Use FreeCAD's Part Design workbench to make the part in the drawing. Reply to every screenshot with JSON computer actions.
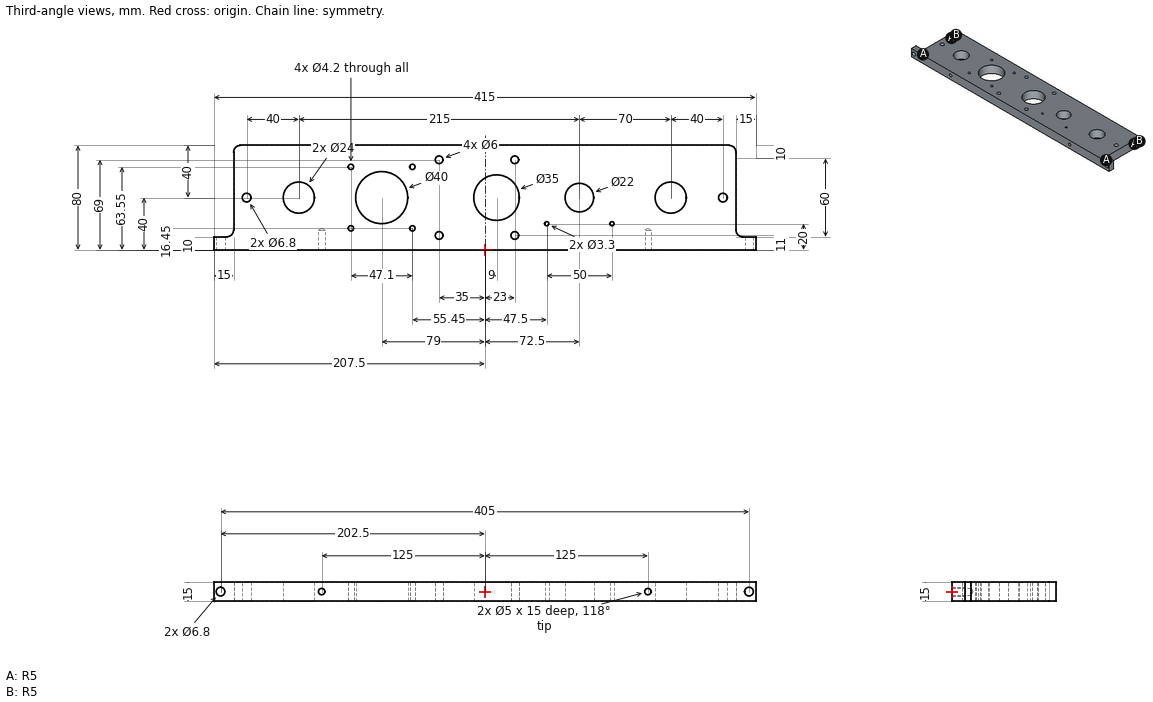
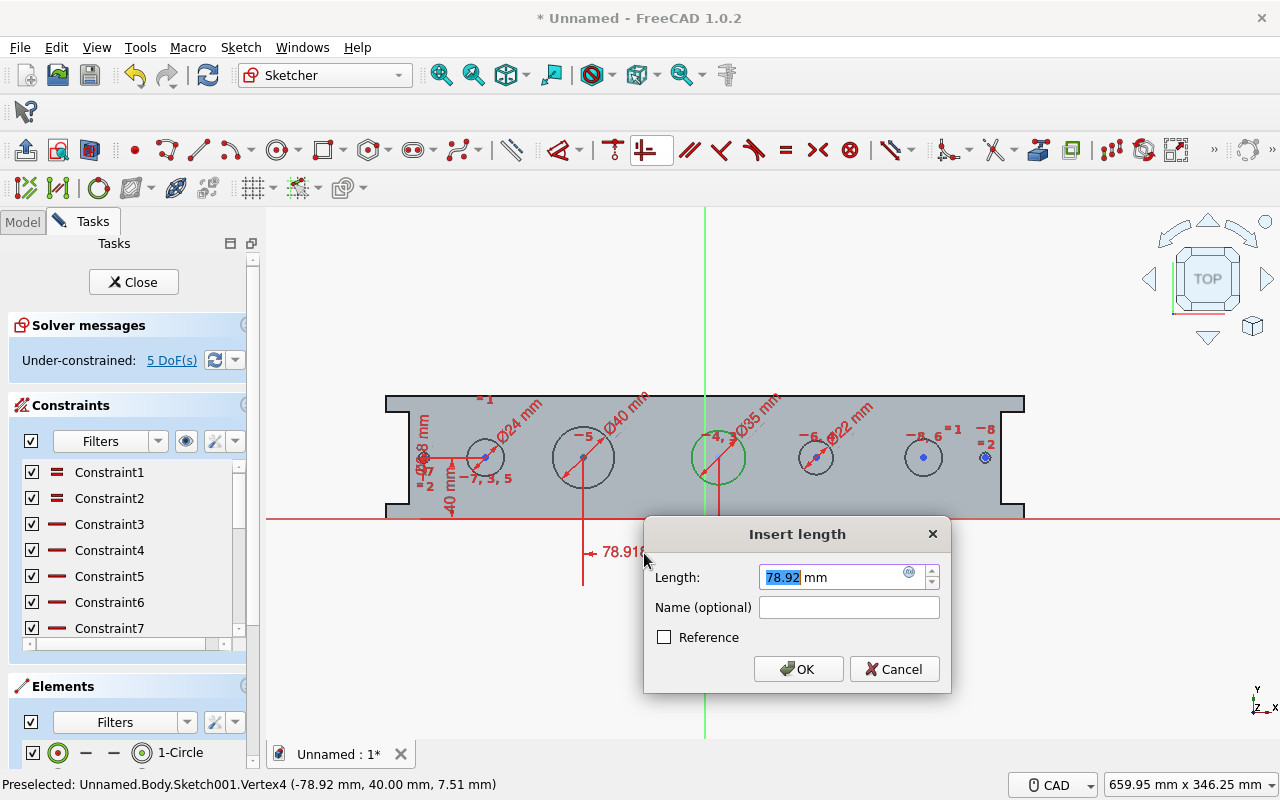
{"action": "type", "text": "79"}
{"action": "key", "text": "Return"}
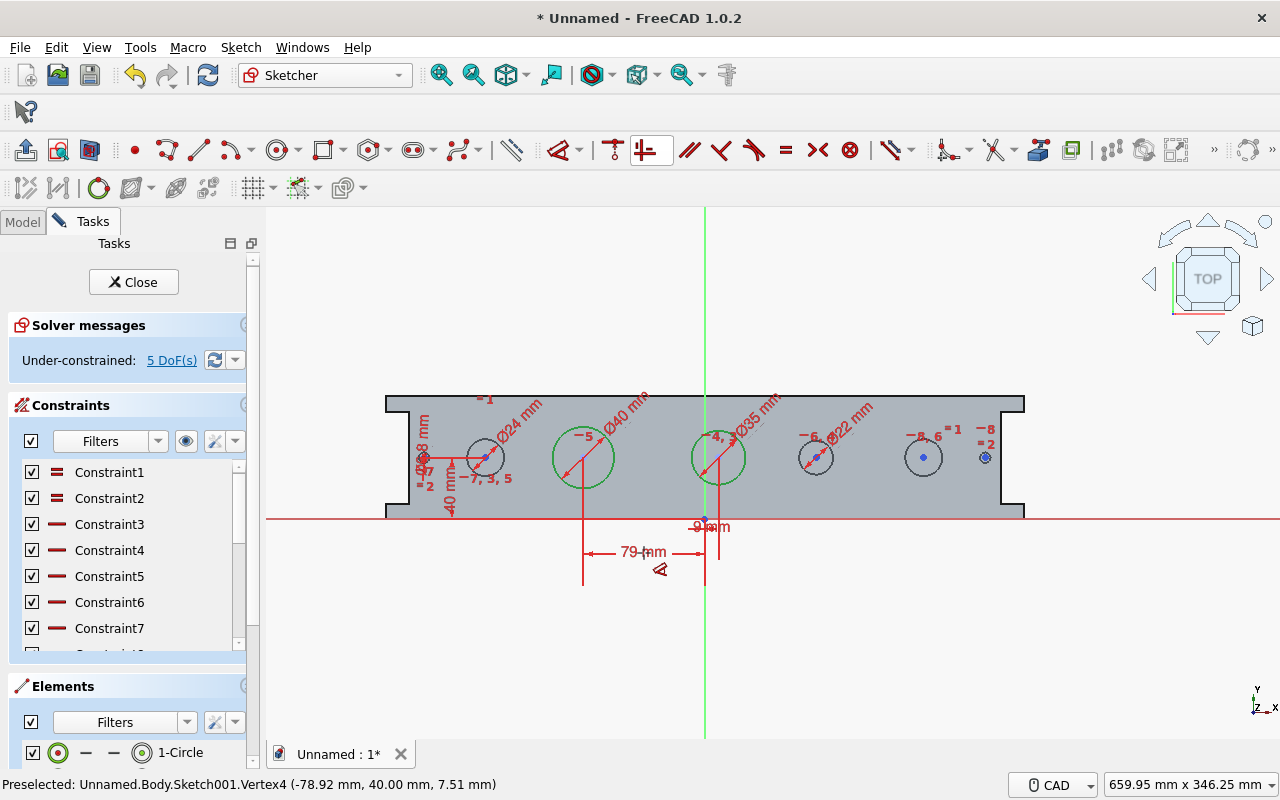
{"action": "left_click", "coordinate": [816, 458]}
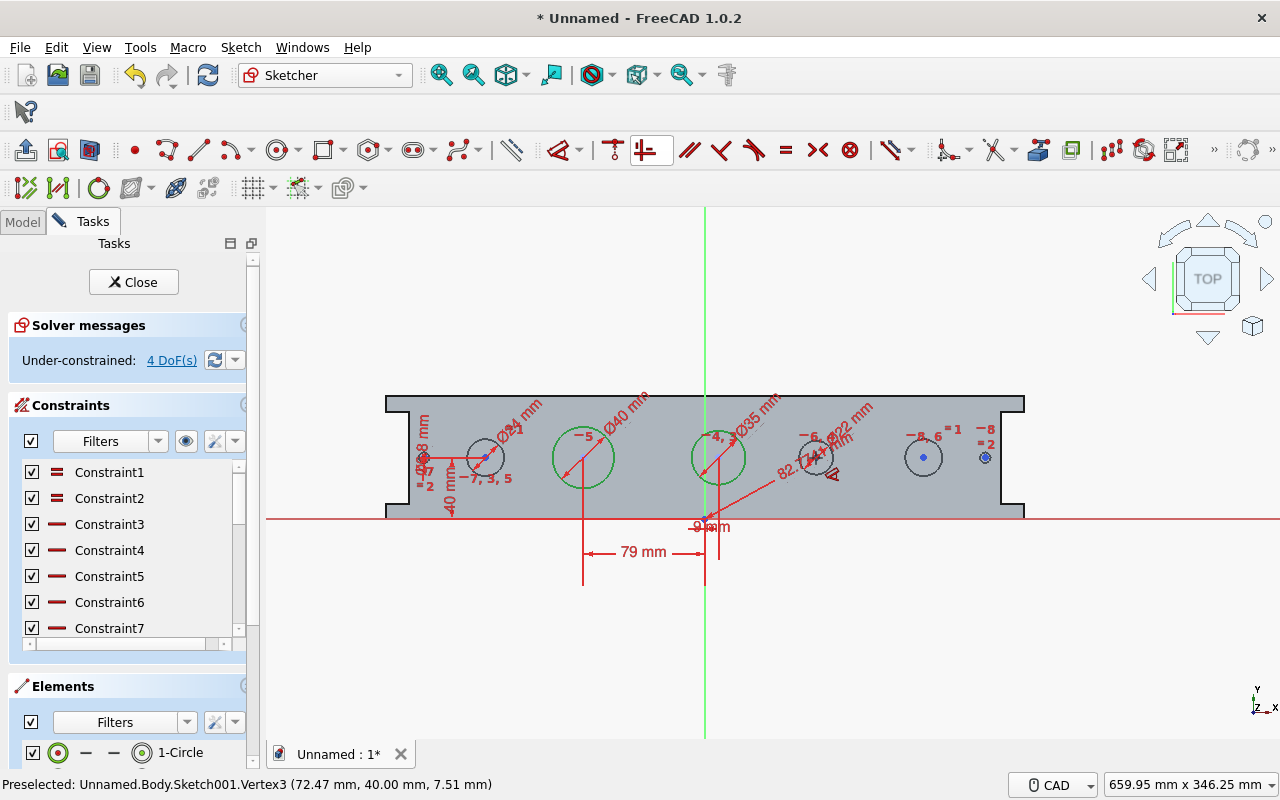
{"action": "left_click", "coordinate": [924, 458]}
{"action": "left_click", "coordinate": [870, 492]}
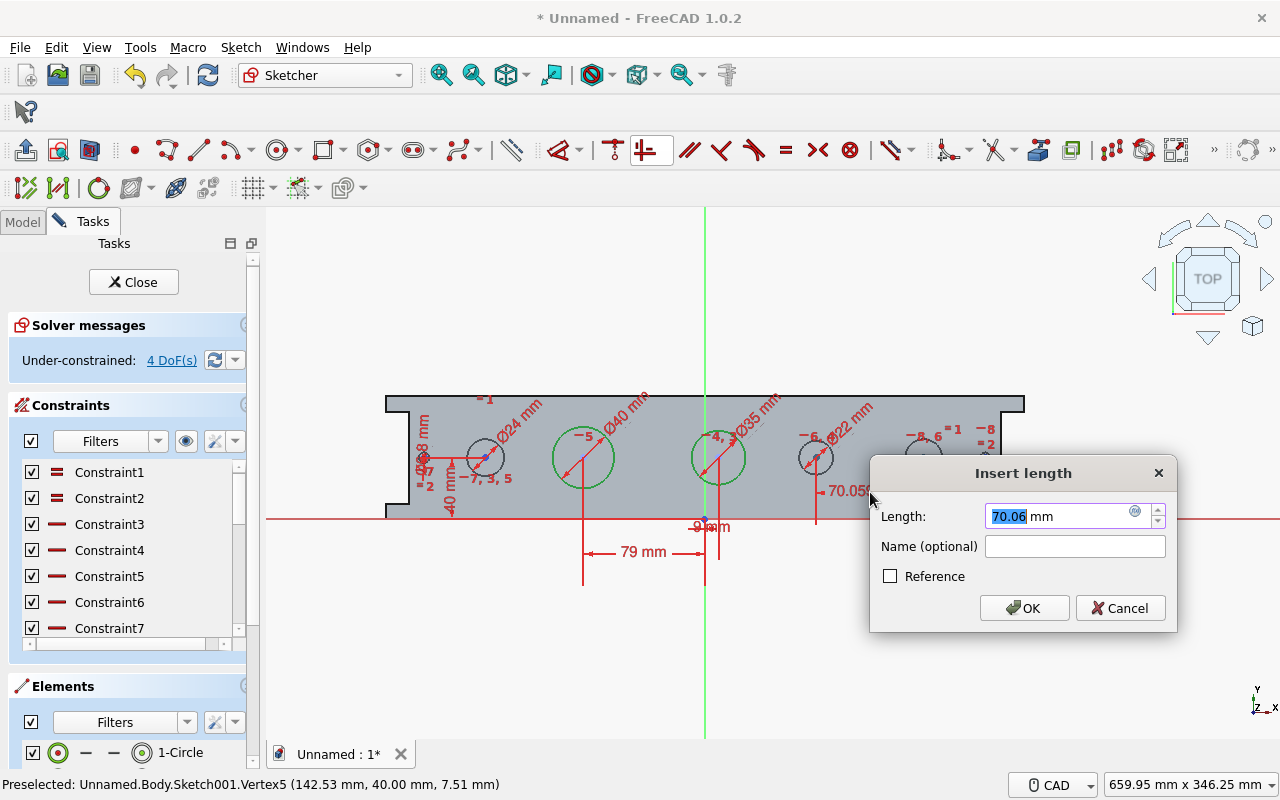
{"action": "type", "text": "70"}
{"action": "key", "text": "Return"}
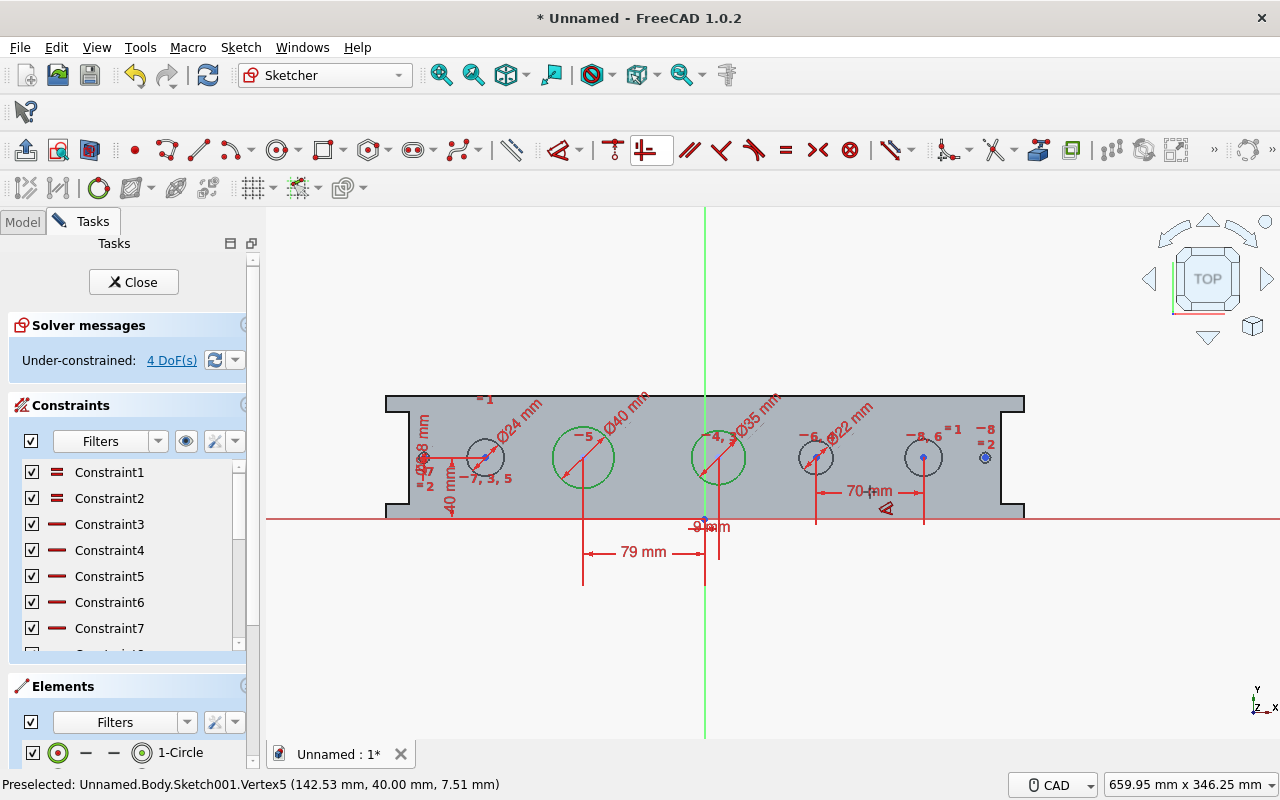
{"action": "left_click", "coordinate": [486, 458]}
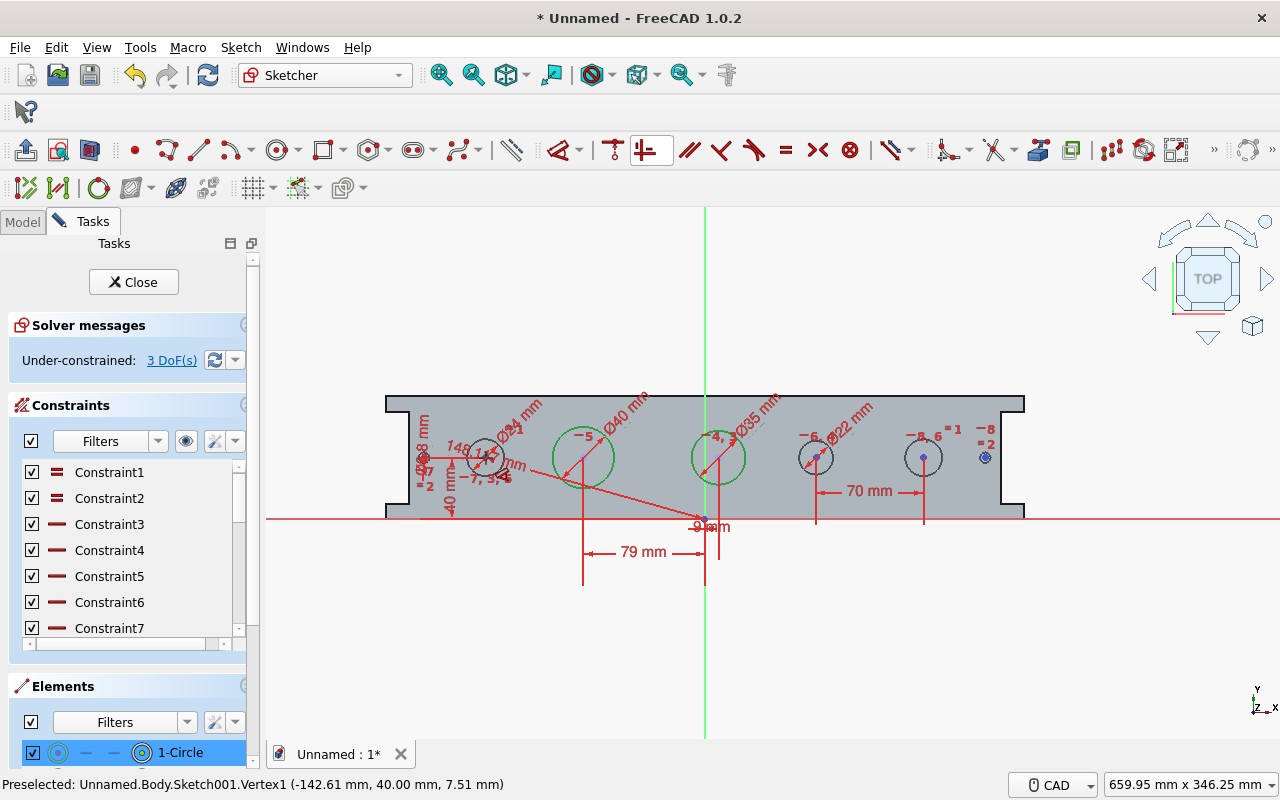
{"action": "left_click", "coordinate": [424, 458]}
{"action": "left_click", "coordinate": [441, 424]}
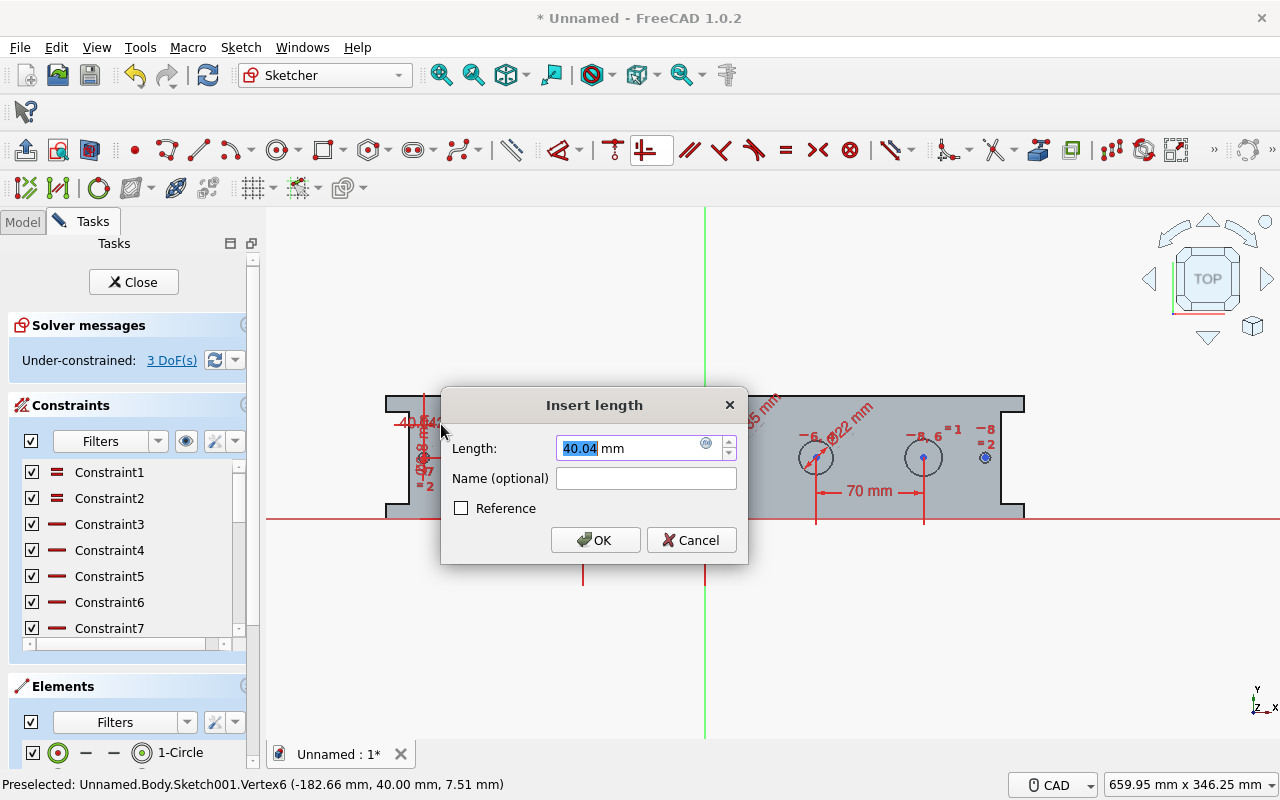
{"action": "type", "text": "40"}
{"action": "key", "text": "Return"}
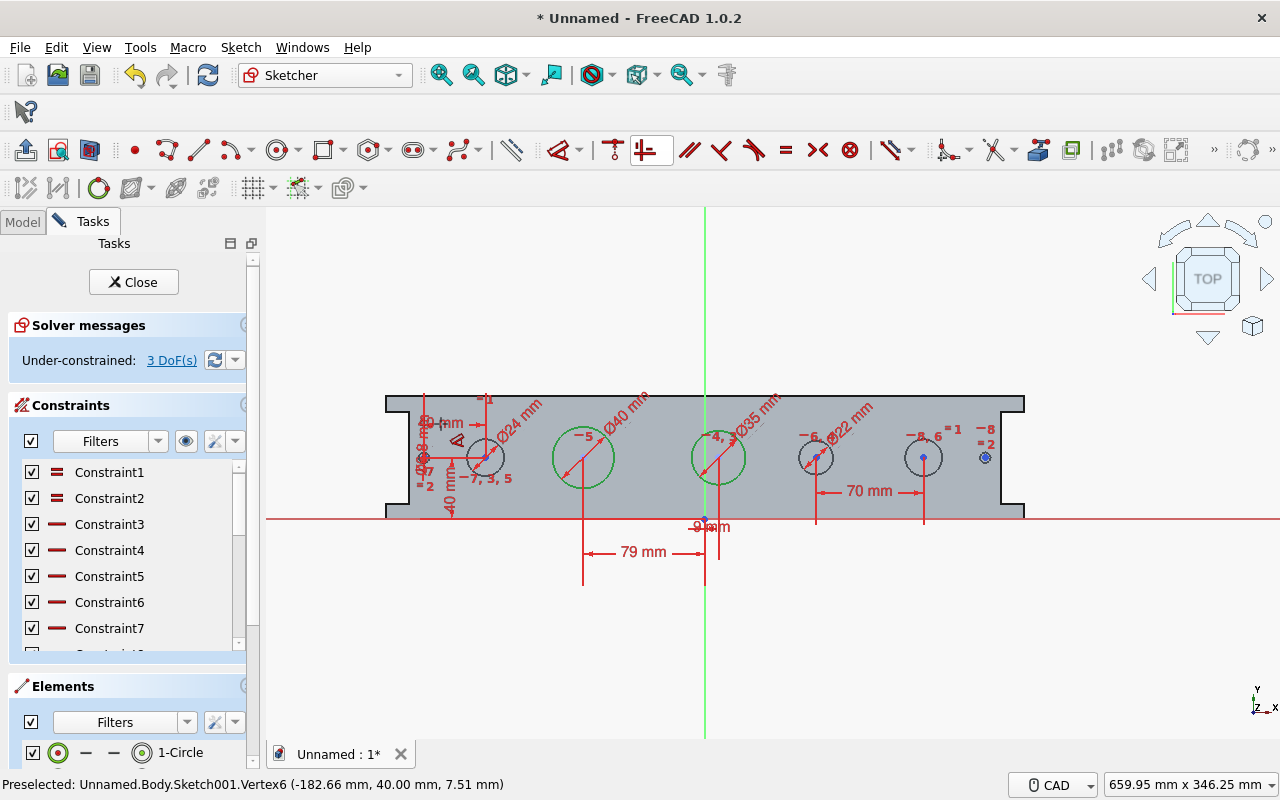
{"action": "left_click", "coordinate": [924, 458]}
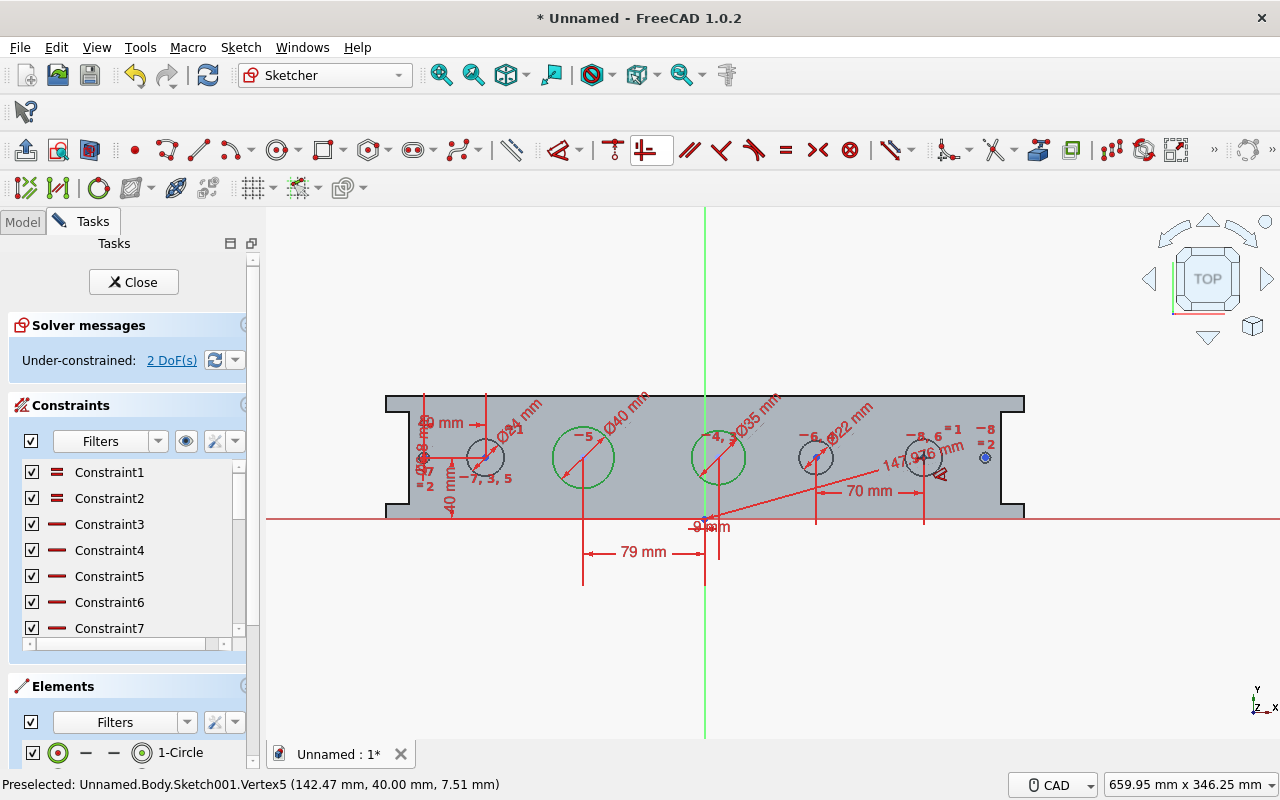
{"action": "left_click", "coordinate": [985, 458]}
{"action": "left_click", "coordinate": [954, 424]}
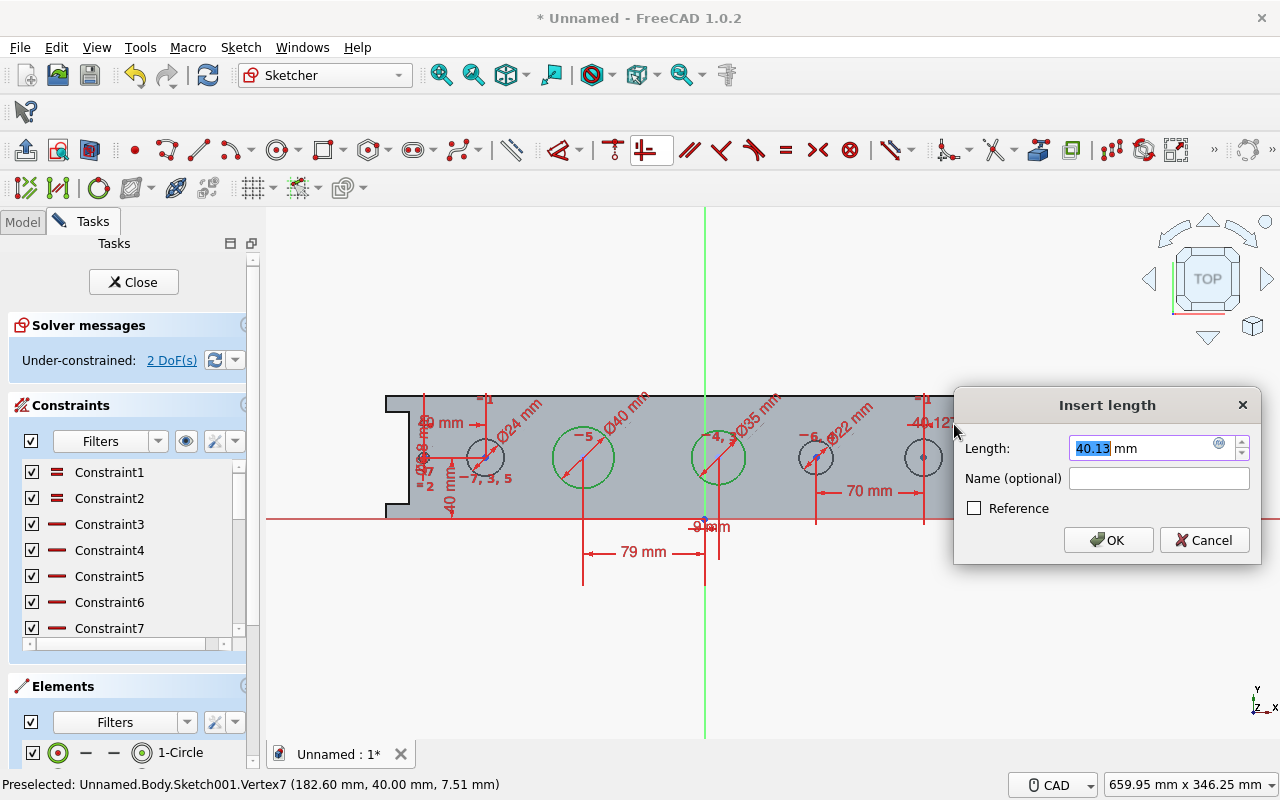
{"action": "type", "text": "40"}
{"action": "key", "text": "Return"}